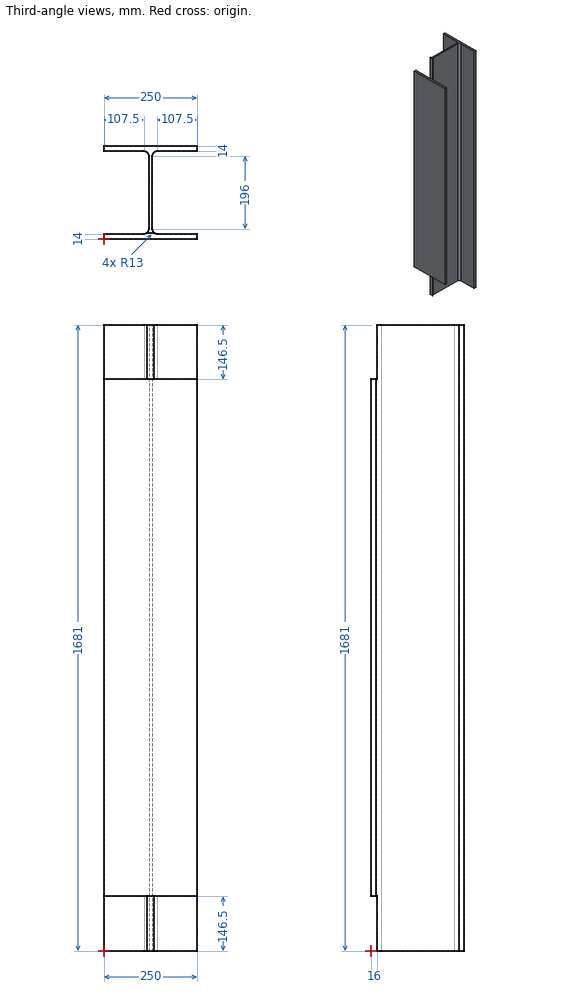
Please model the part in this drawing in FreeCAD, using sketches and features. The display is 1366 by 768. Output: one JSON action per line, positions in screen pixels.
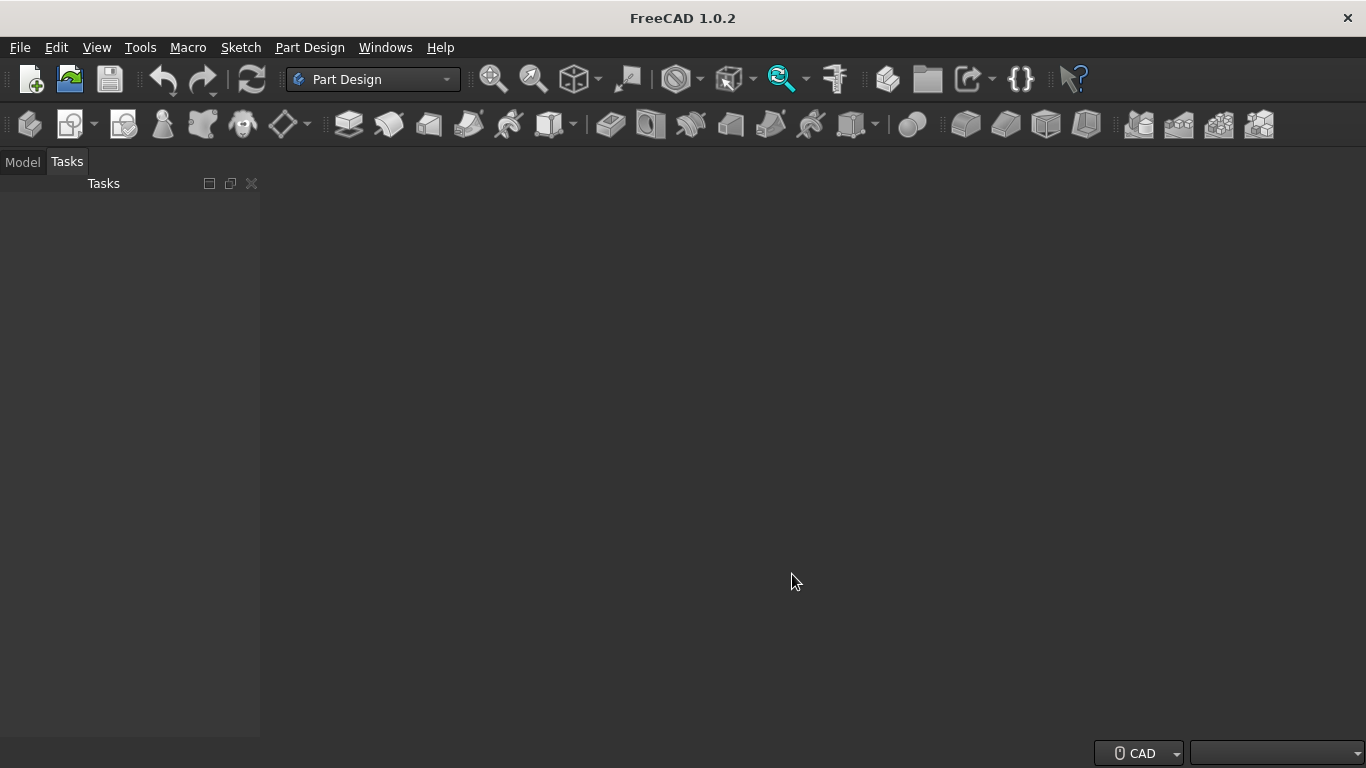
{"action": "left_click", "coordinate": [30, 80]}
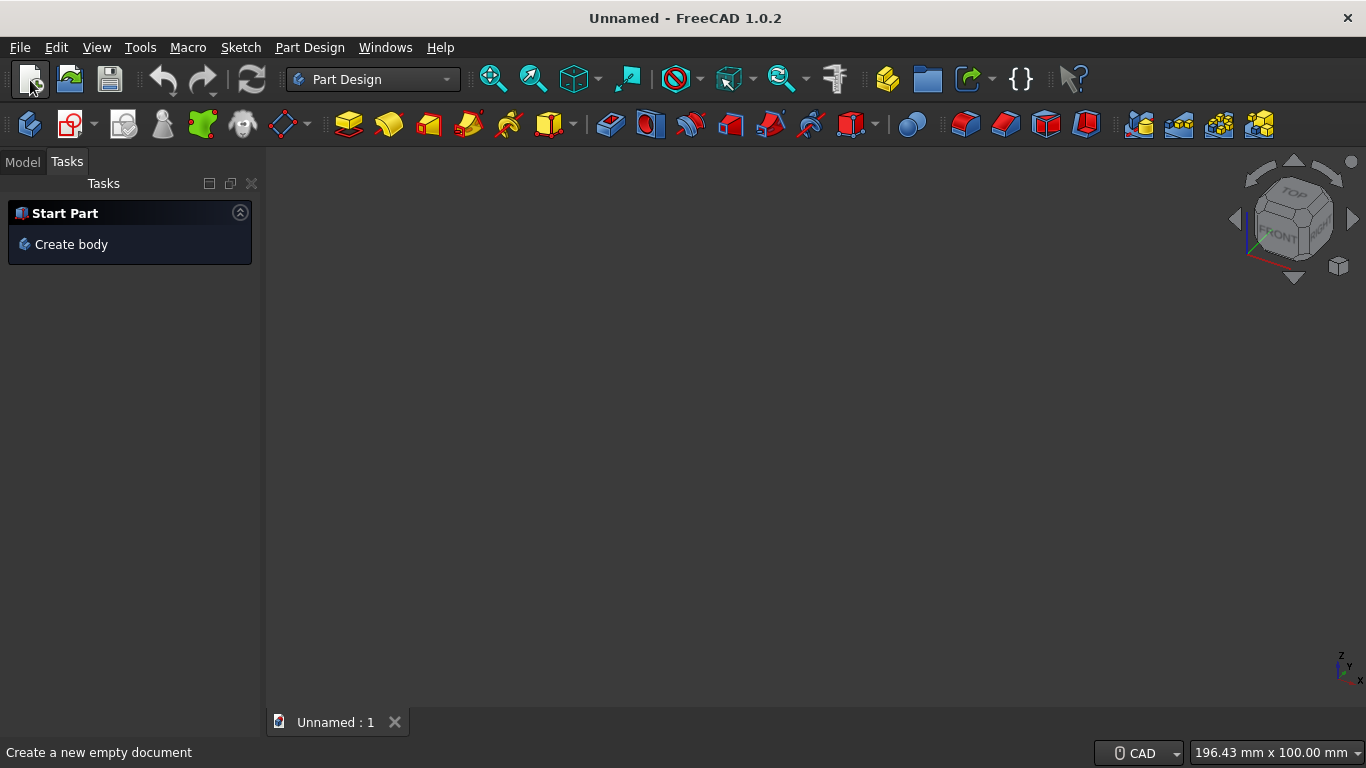
{"action": "left_click", "coordinate": [70, 124]}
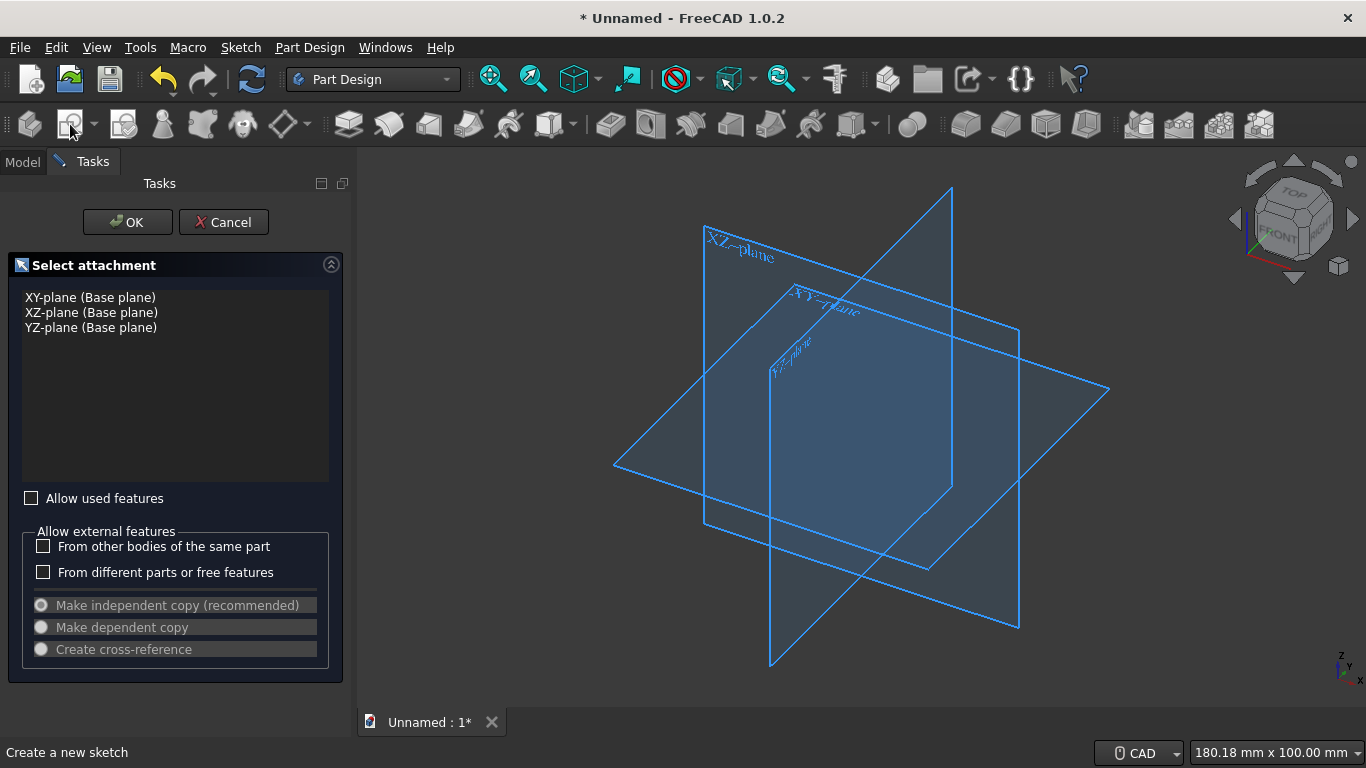
{"action": "left_click", "coordinate": [82, 298]}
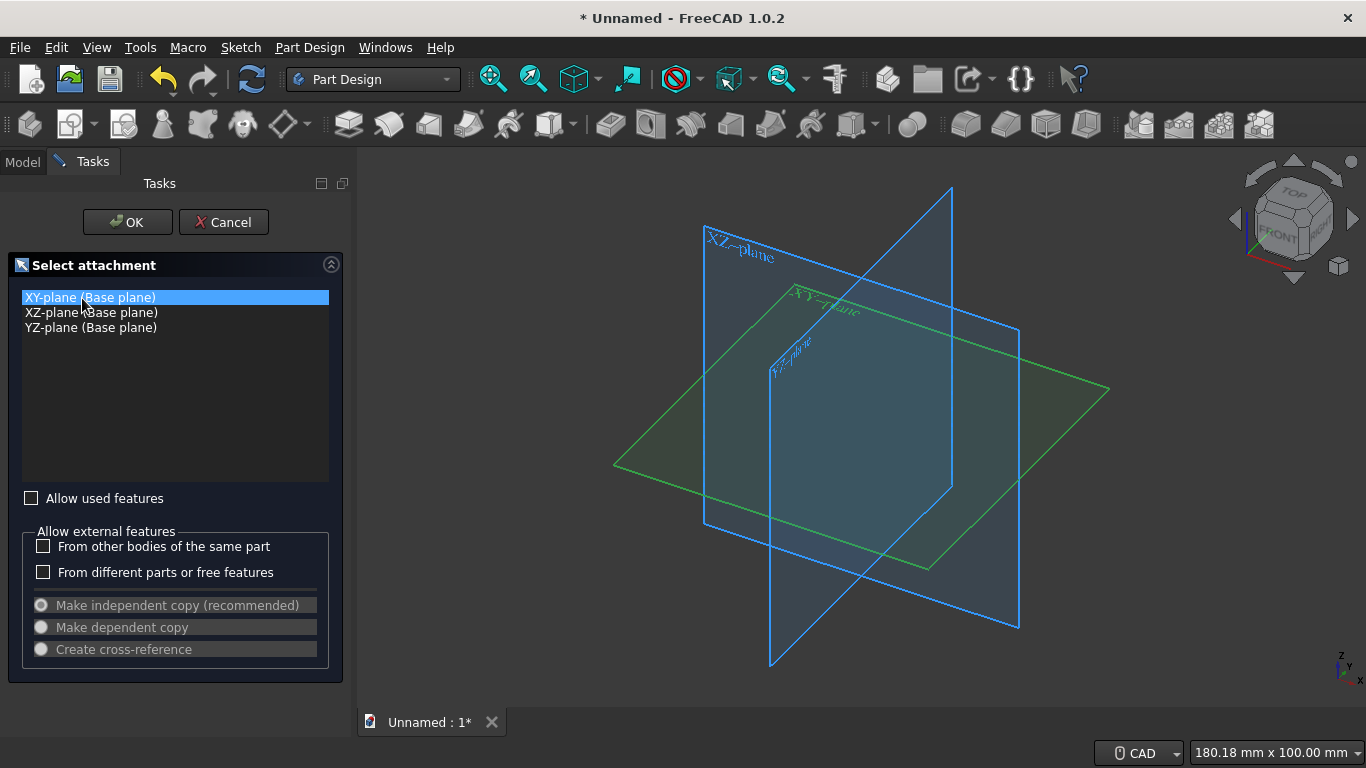
{"action": "left_click", "coordinate": [128, 222]}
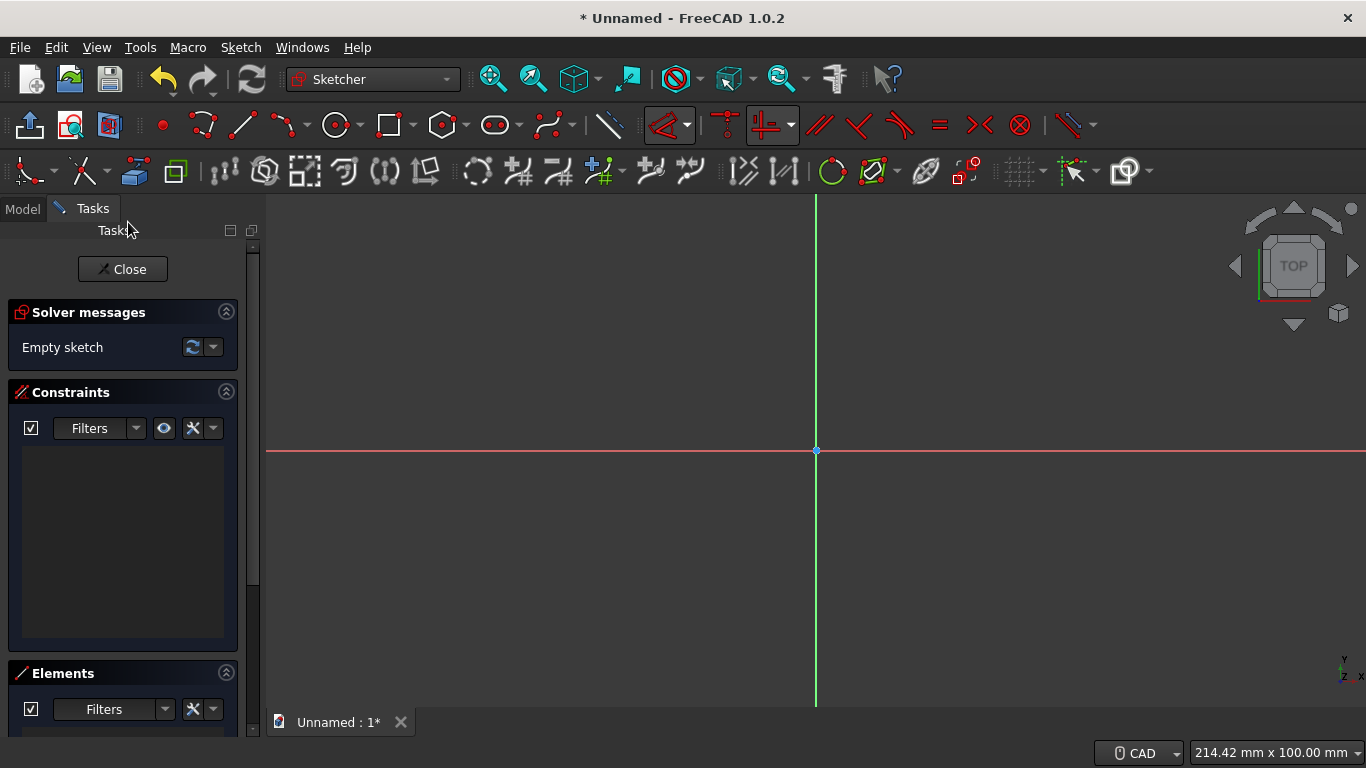
{"action": "scroll", "coordinate": [515, 660], "scroll_direction": "down", "scroll_amount": 7}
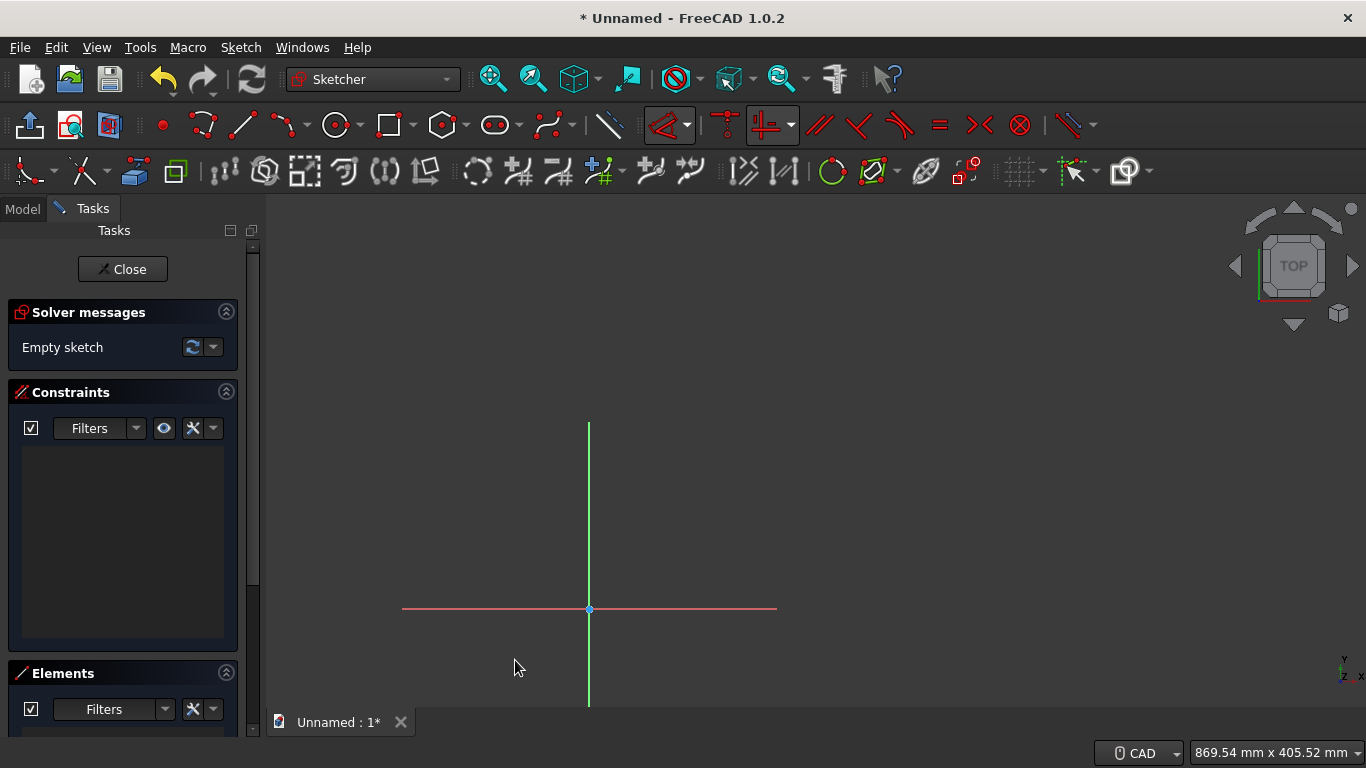
{"action": "left_click", "coordinate": [244, 126]}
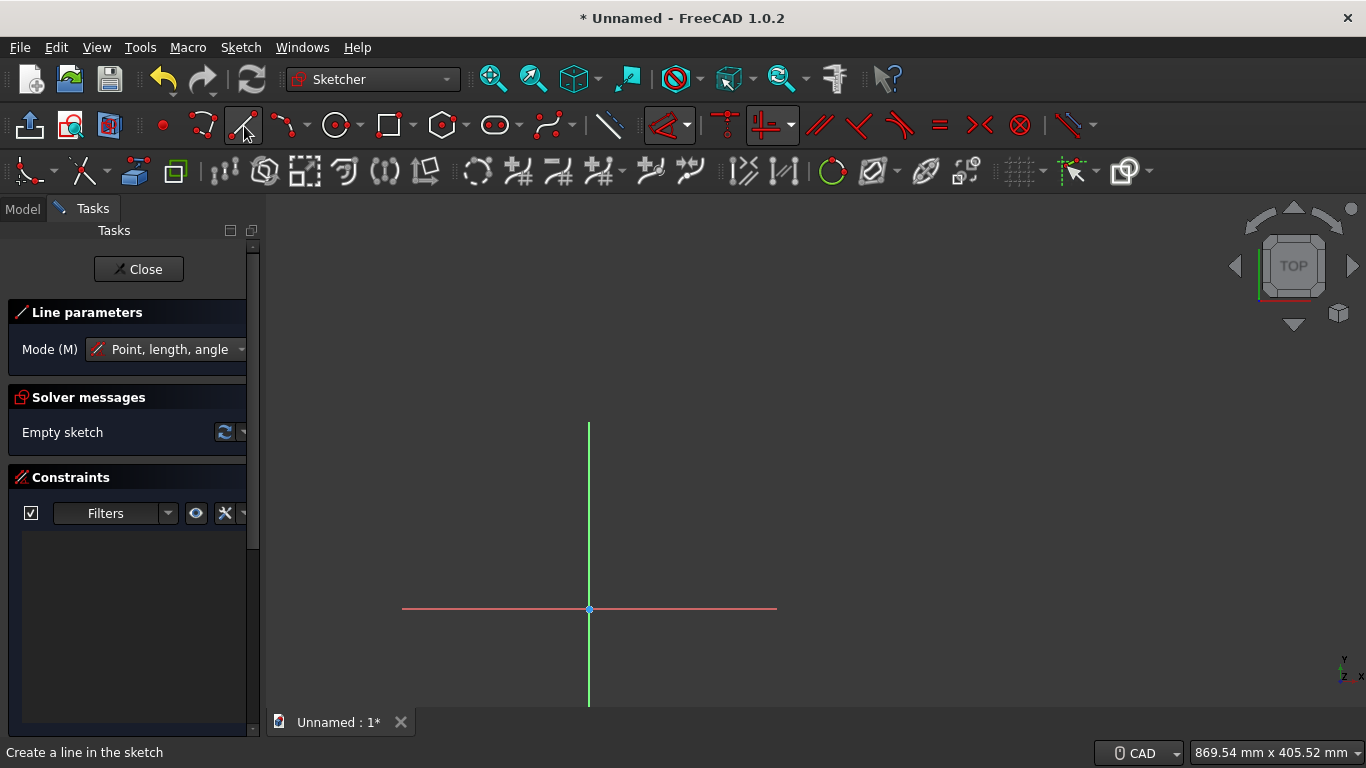
{"action": "left_click", "coordinate": [753, 575]}
{"action": "left_click", "coordinate": [753, 327]}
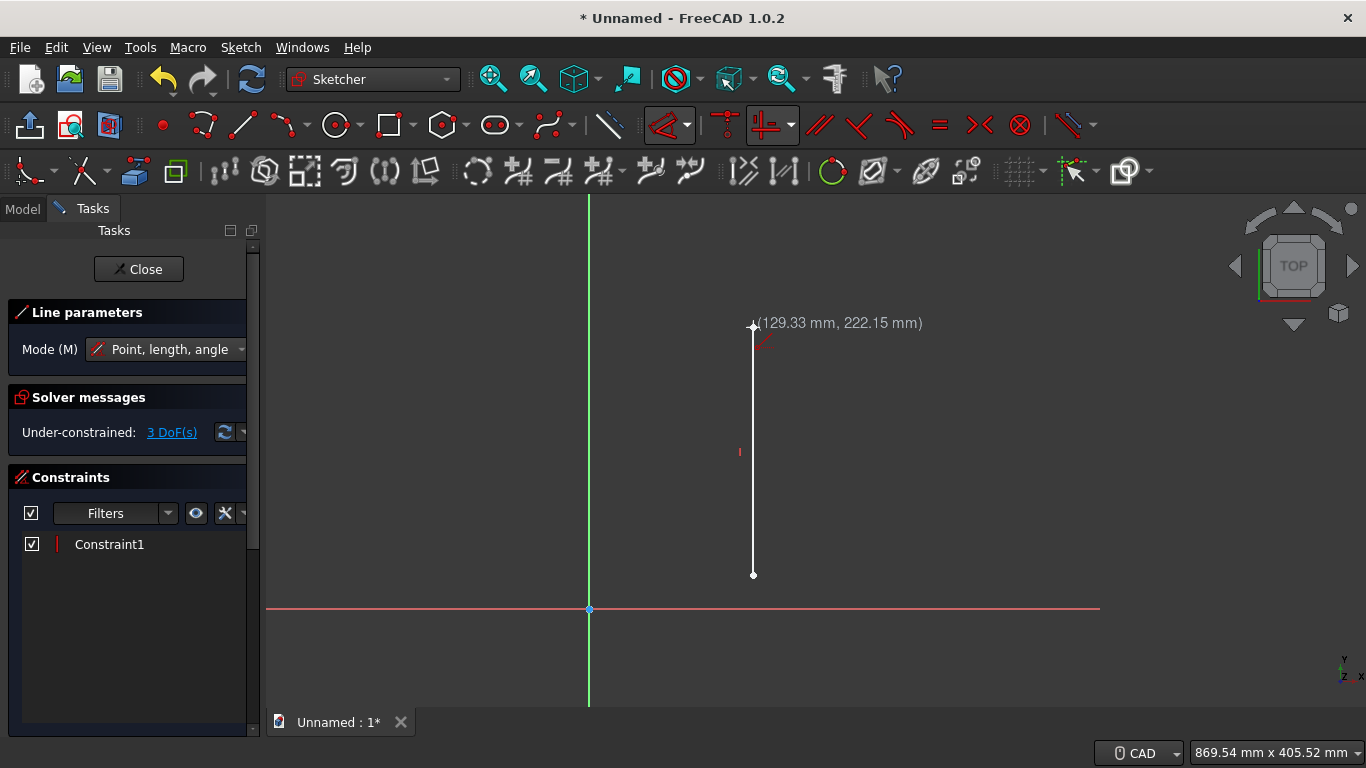
{"action": "left_click", "coordinate": [204, 126]}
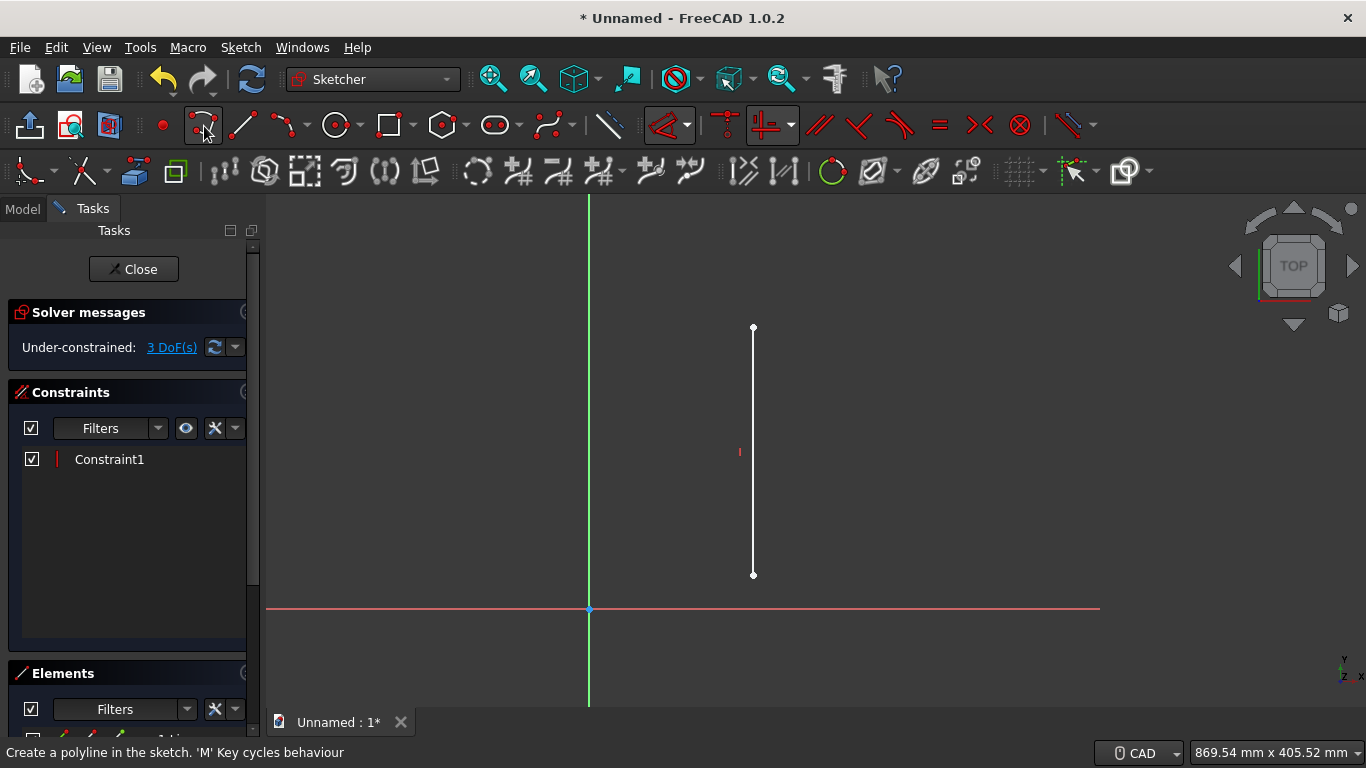
{"action": "left_click", "coordinate": [770, 310]}
{"action": "left_click", "coordinate": [906, 310]}
{"action": "left_click", "coordinate": [906, 293]}
{"action": "left_click", "coordinate": [589, 293]}
{"action": "left_click", "coordinate": [598, 310]}
{"action": "left_click", "coordinate": [725, 310]}
{"action": "right_click", "coordinate": [725, 310]}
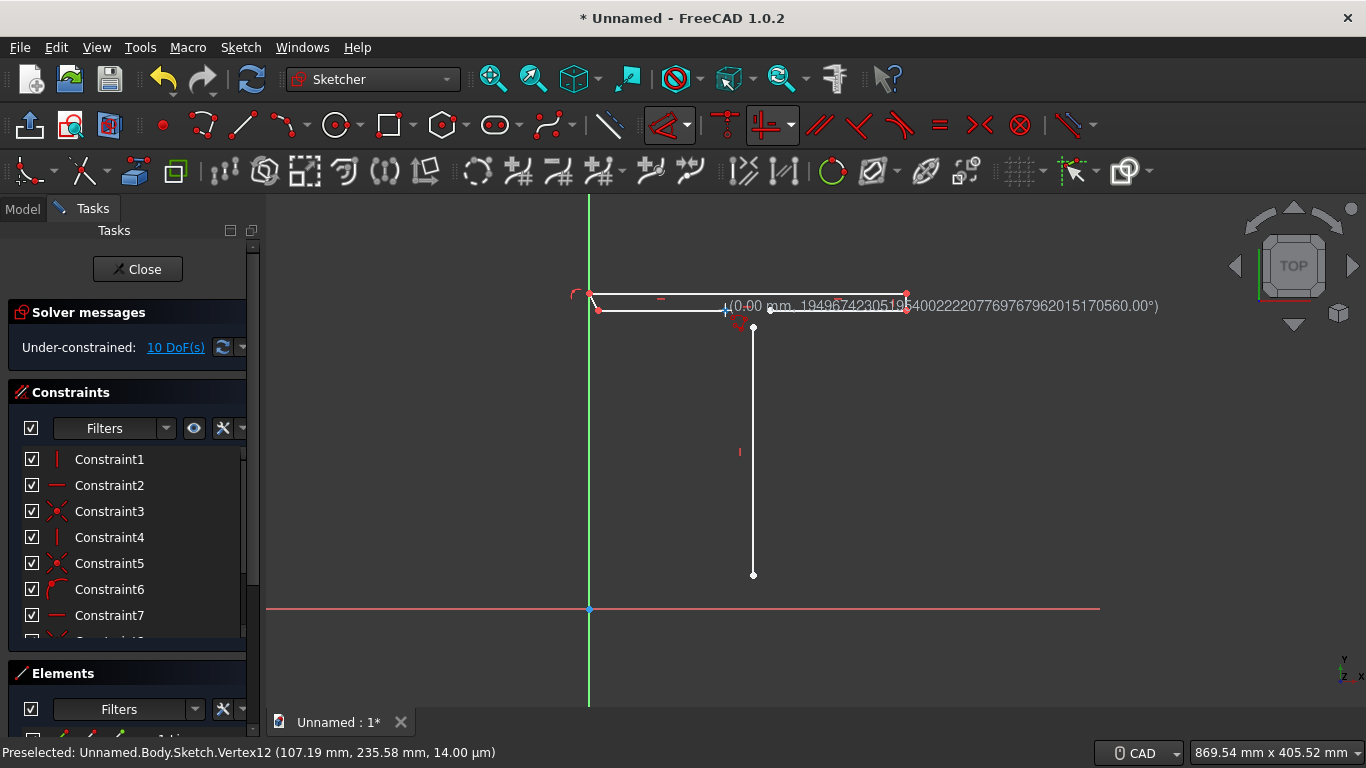
{"action": "left_click", "coordinate": [244, 126]}